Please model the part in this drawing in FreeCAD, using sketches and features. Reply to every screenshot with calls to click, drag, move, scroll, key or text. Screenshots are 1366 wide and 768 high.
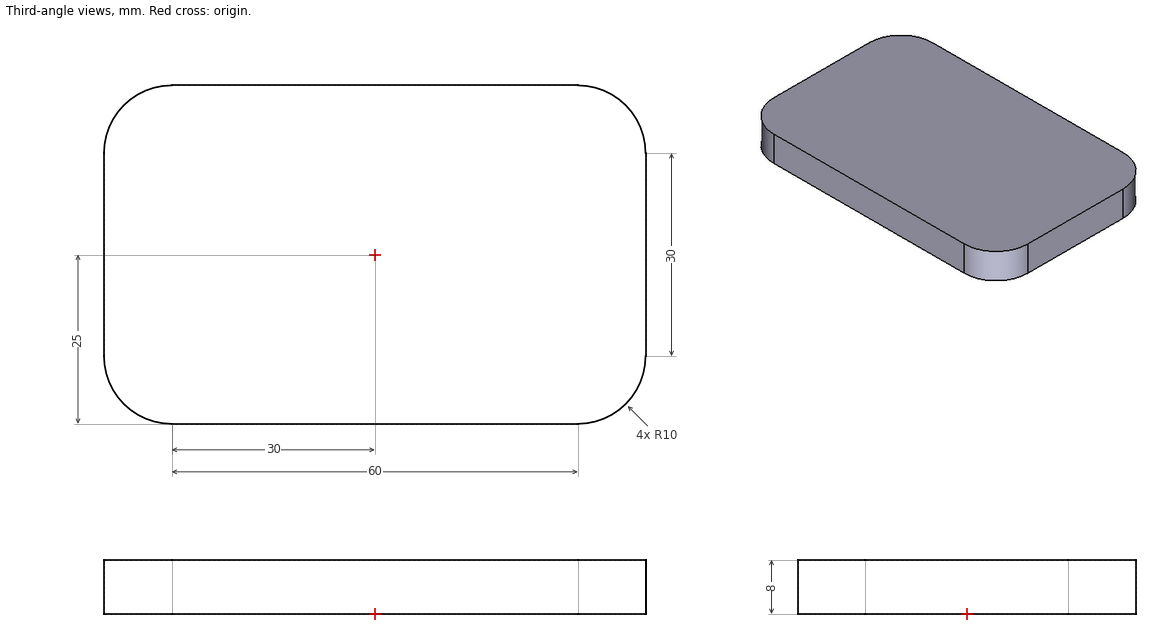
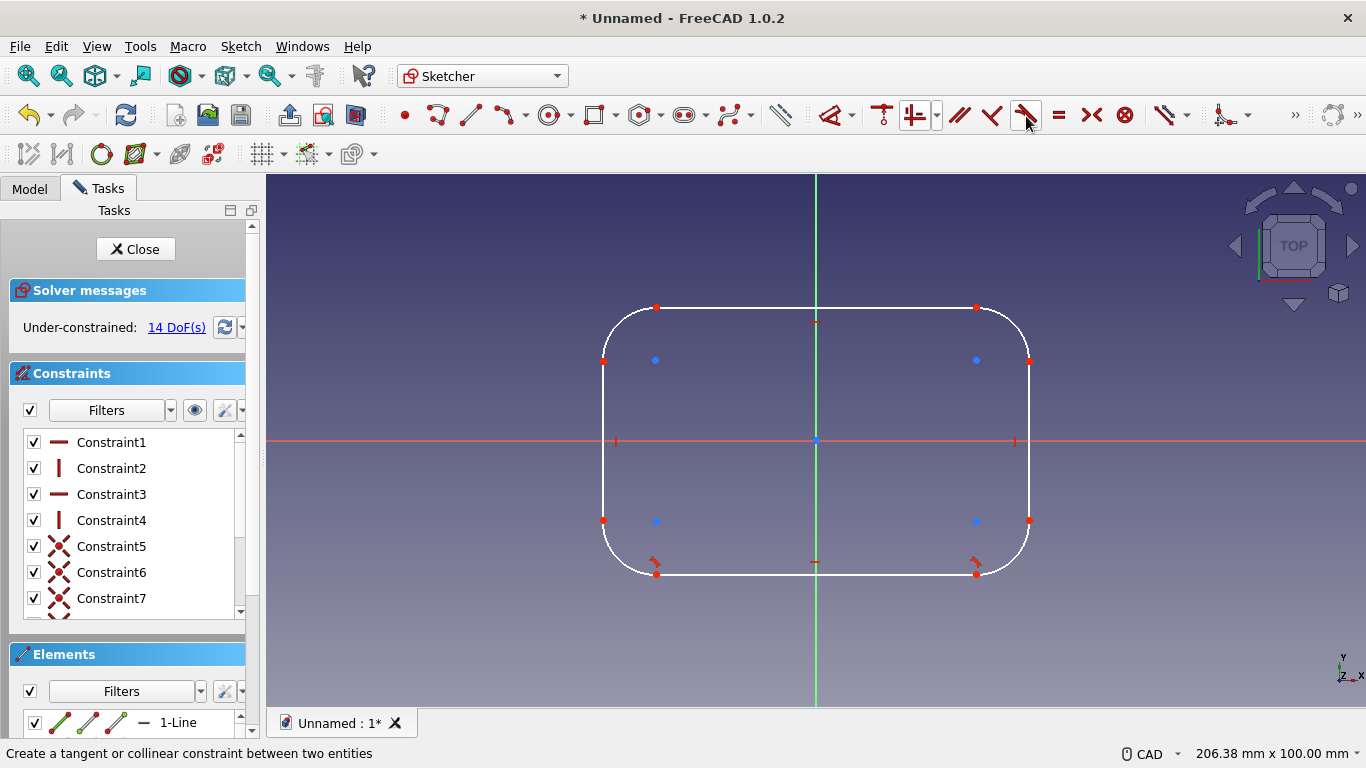
click(1029, 473)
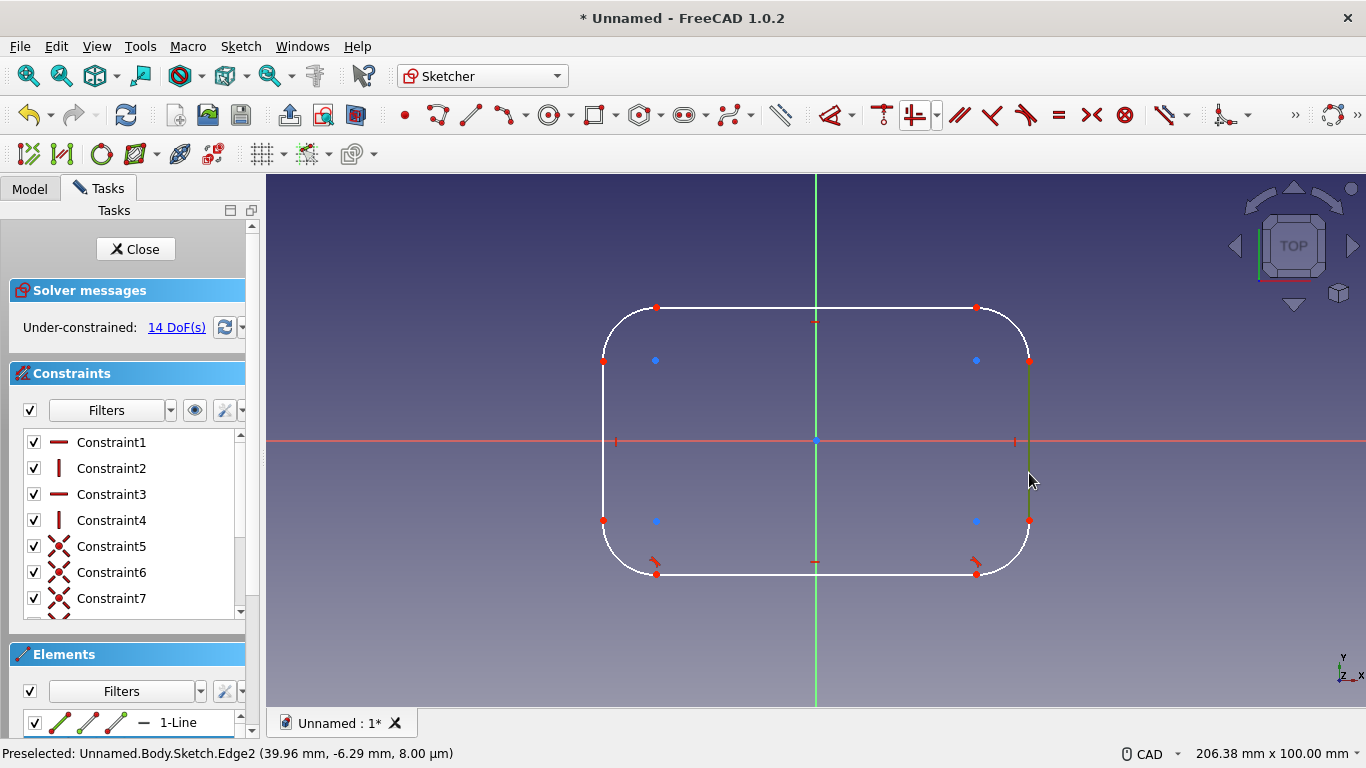
click(1000, 569)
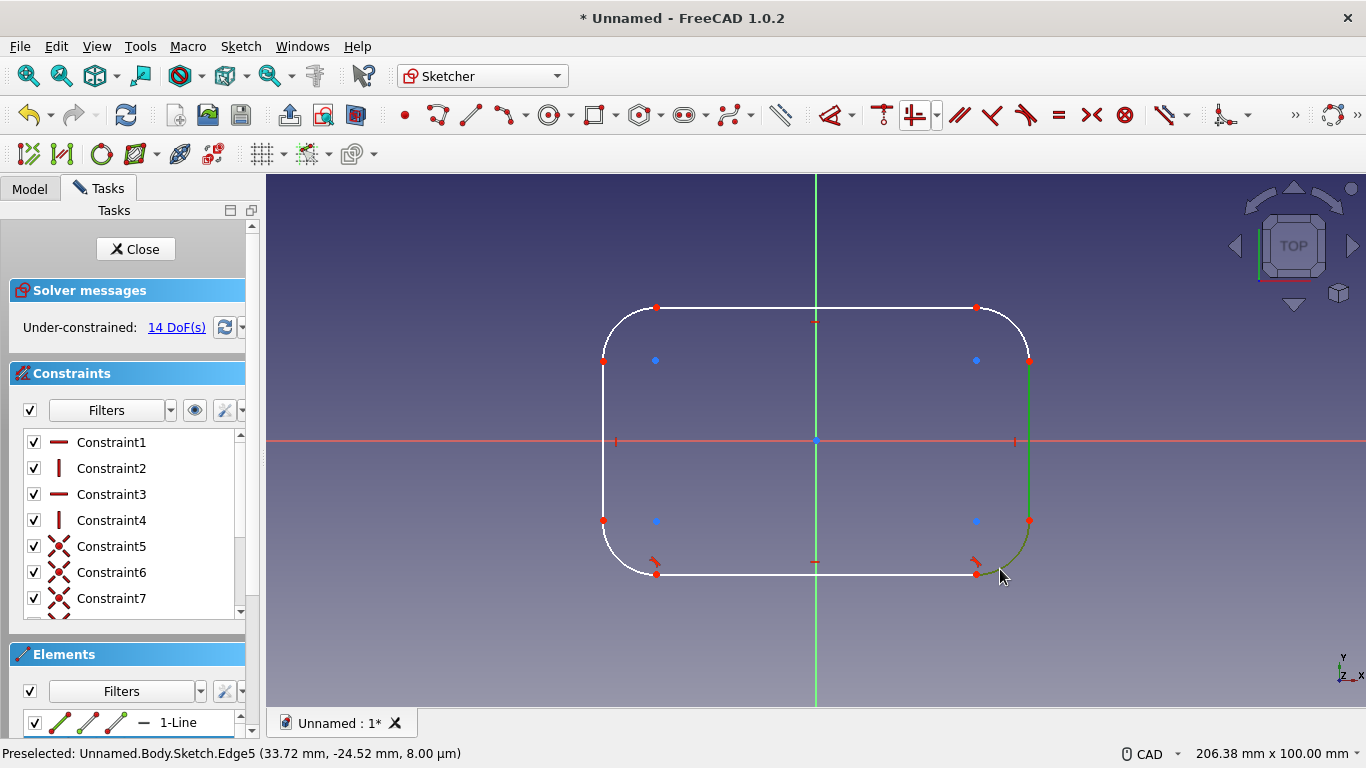
click(1026, 116)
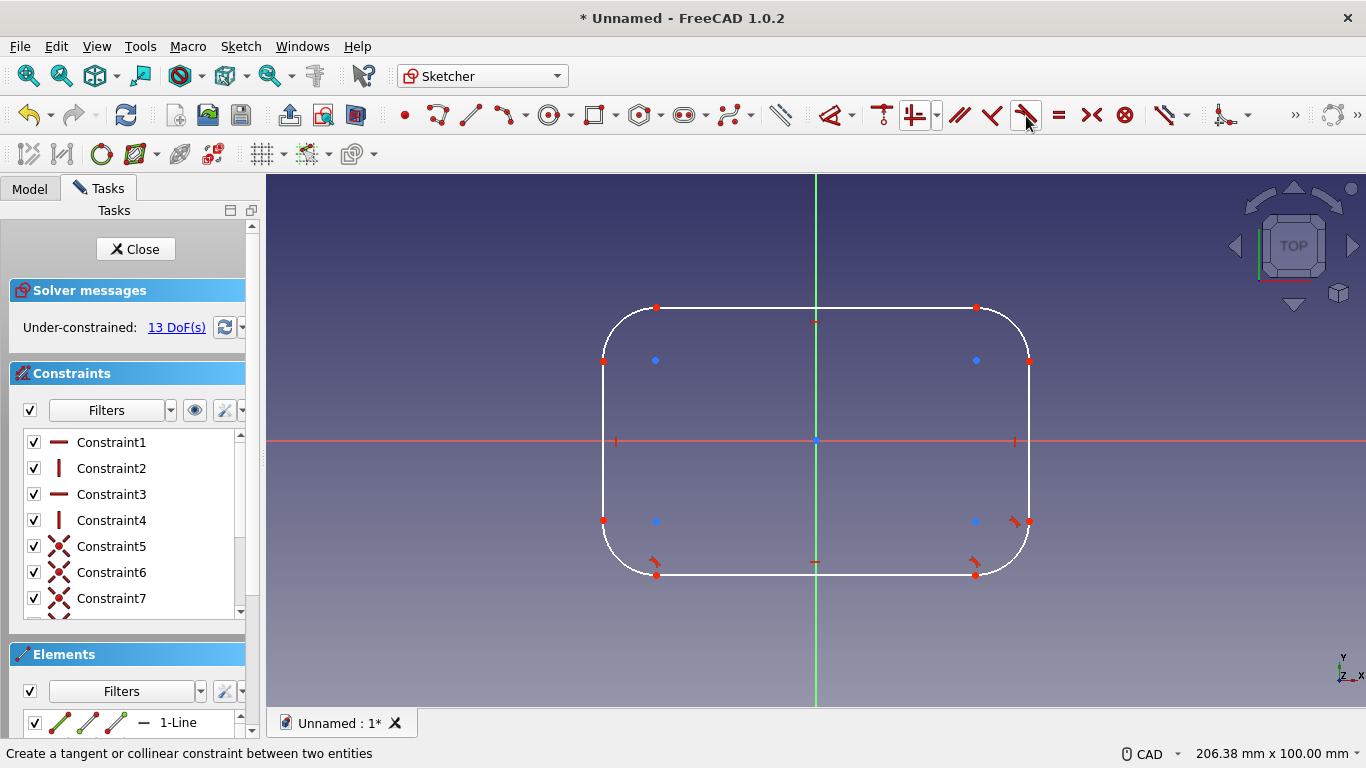
click(1029, 473)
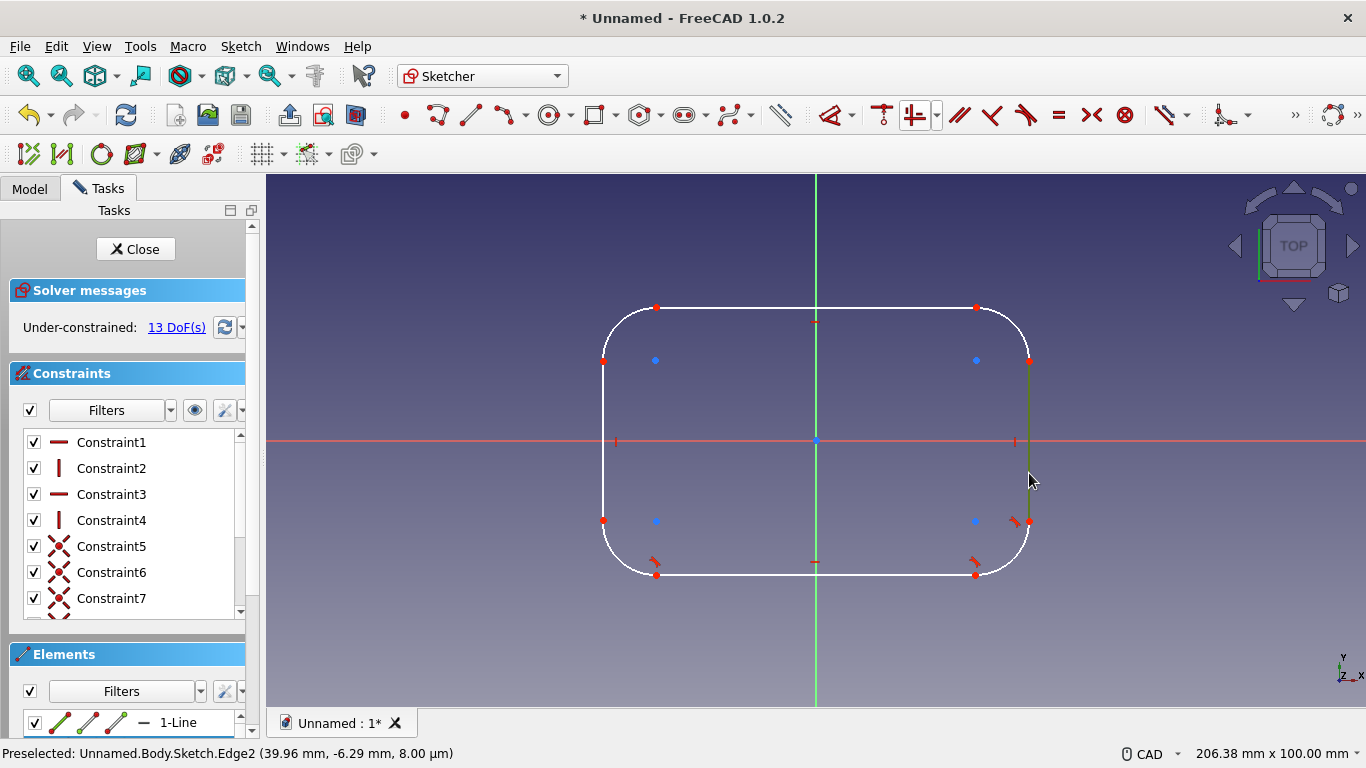
click(1024, 338)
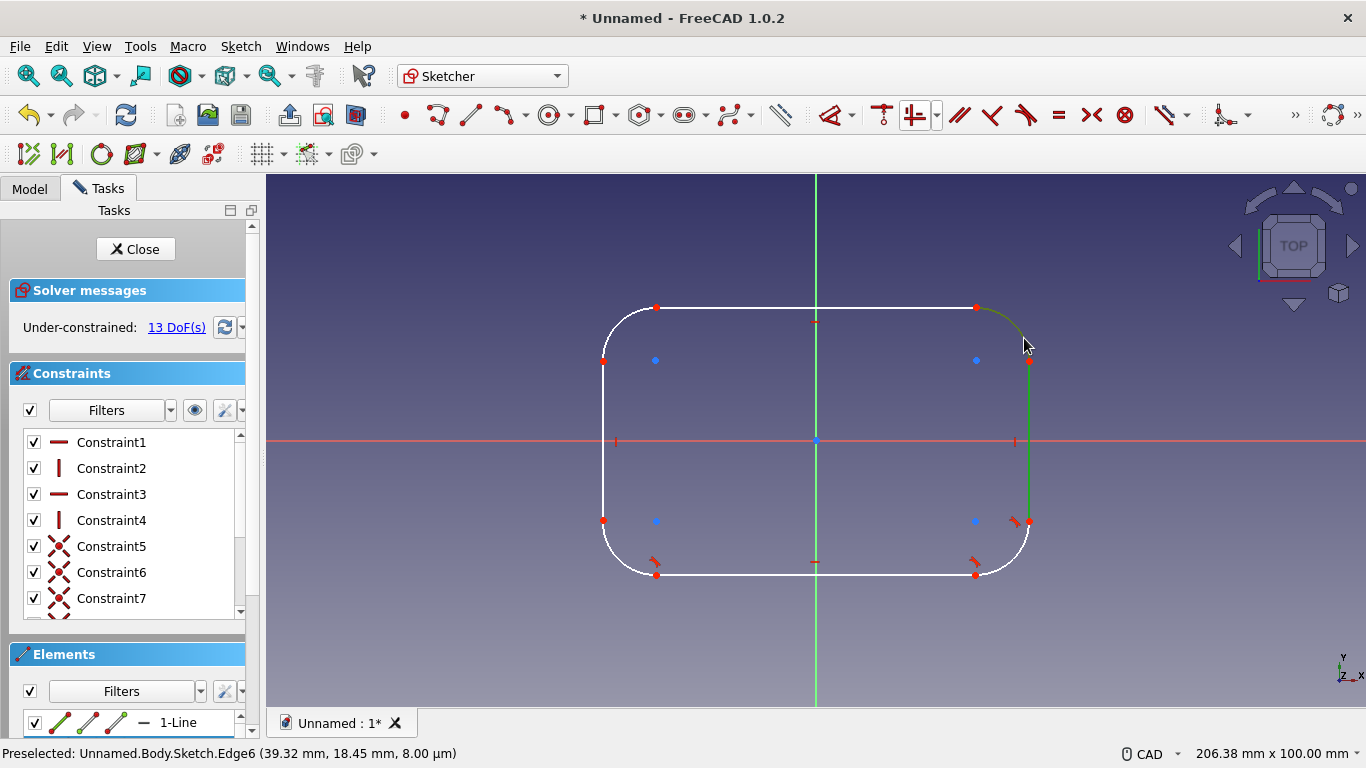
key(t)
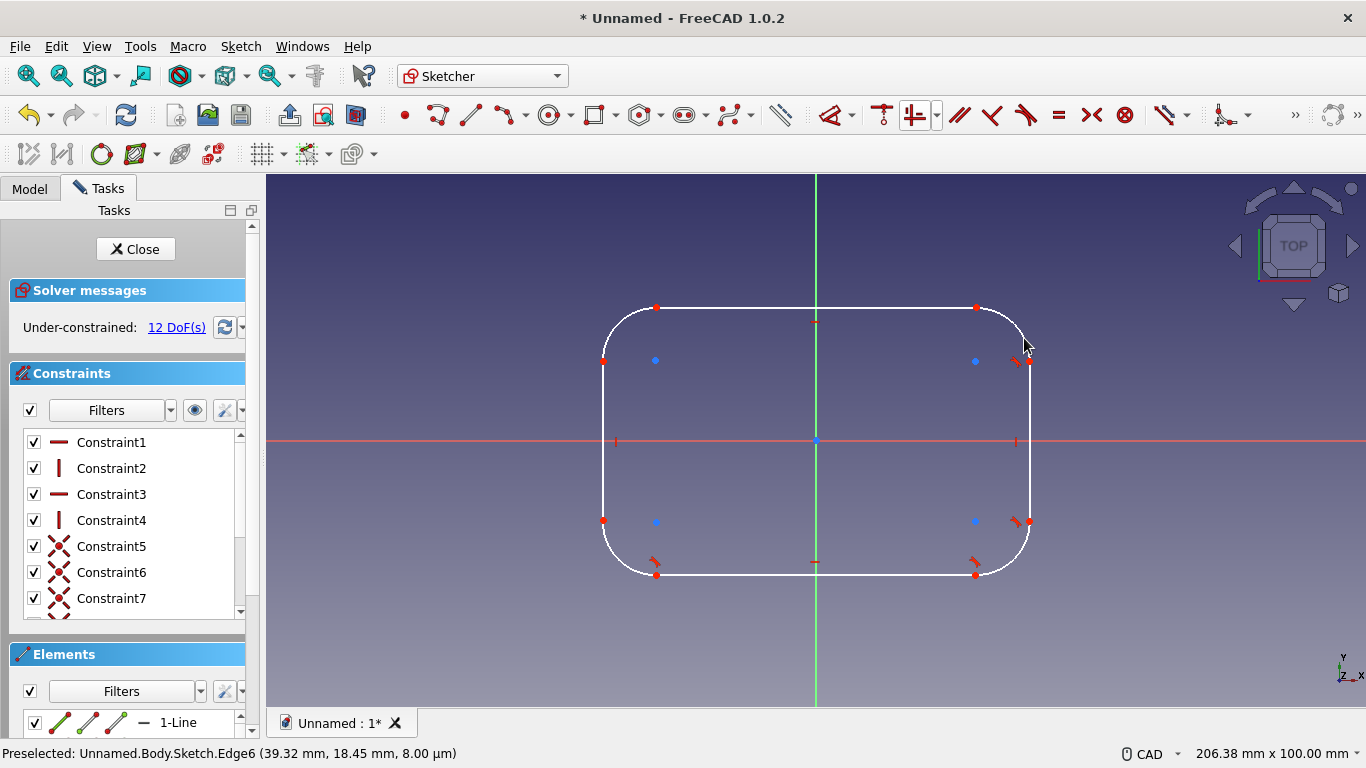
click(880, 308)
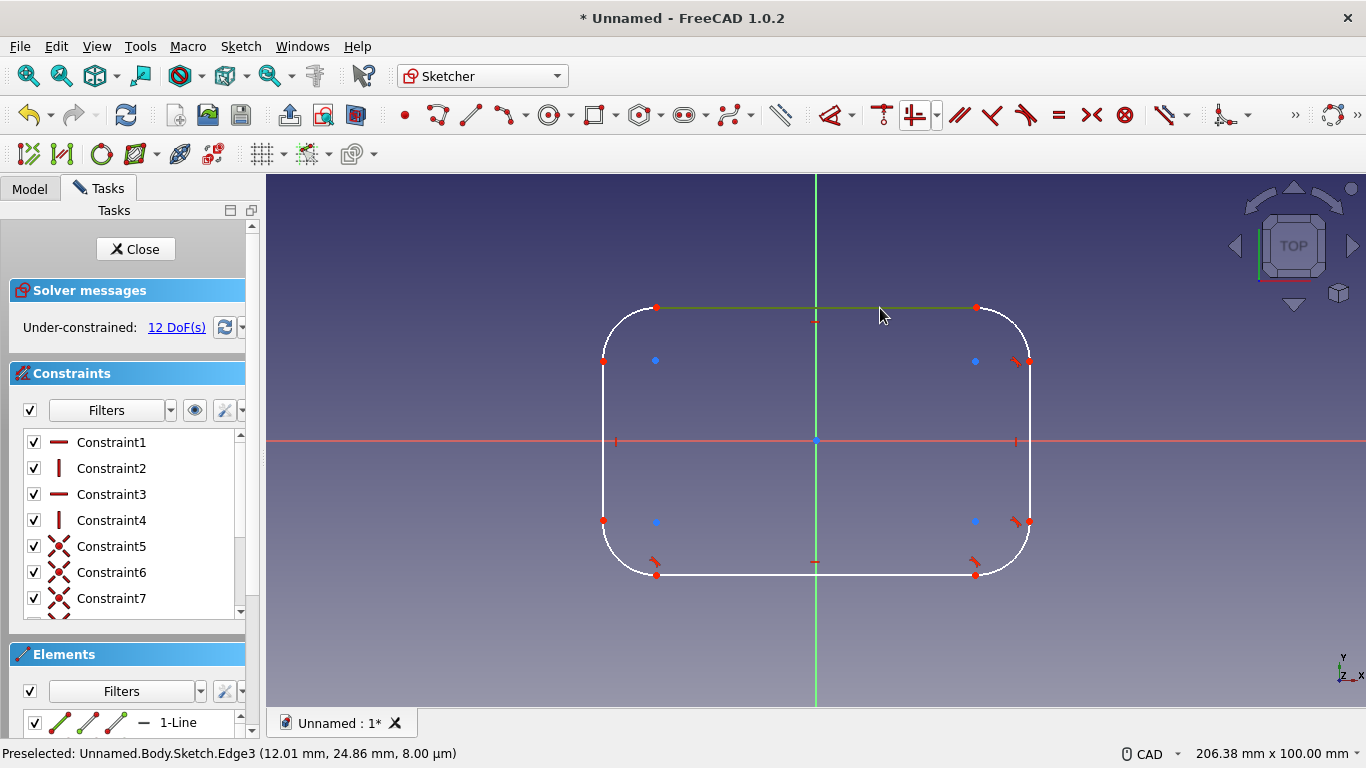
click(1024, 338)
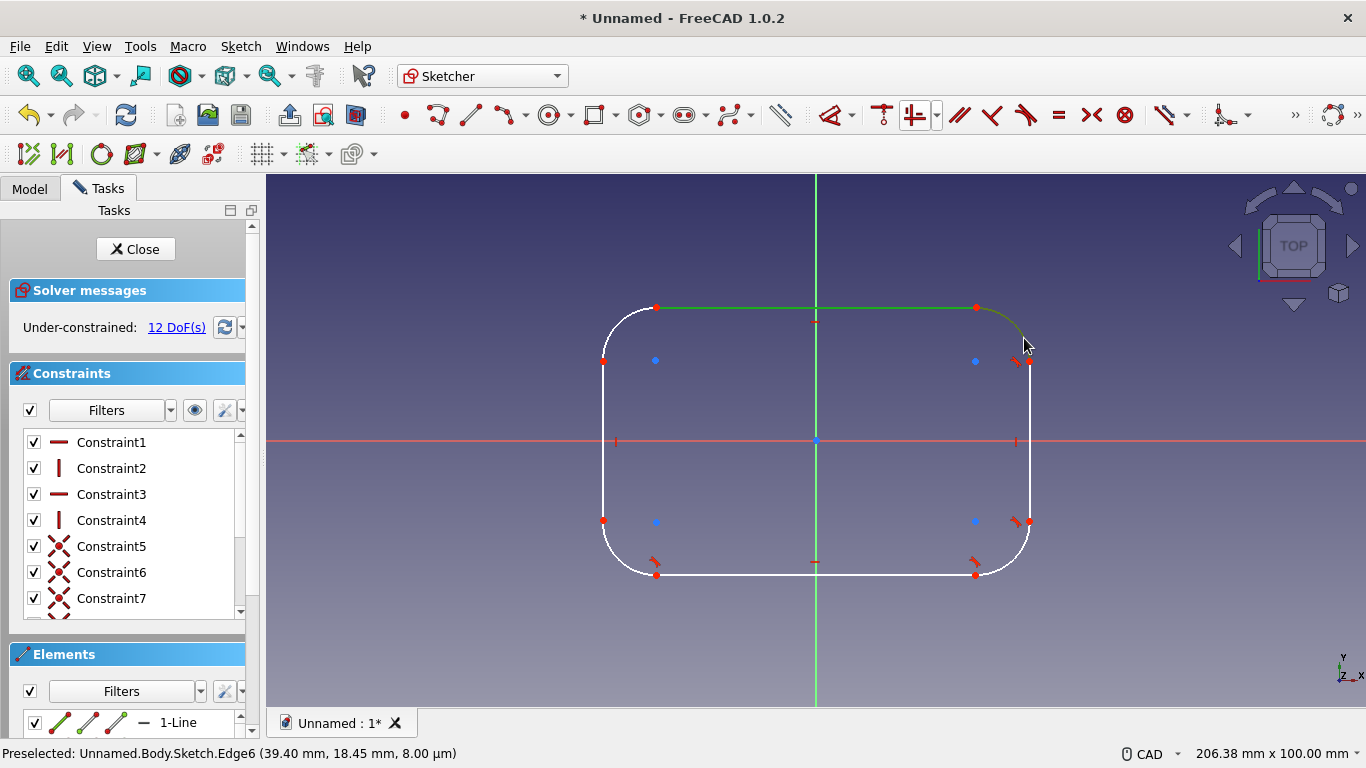
click(1026, 116)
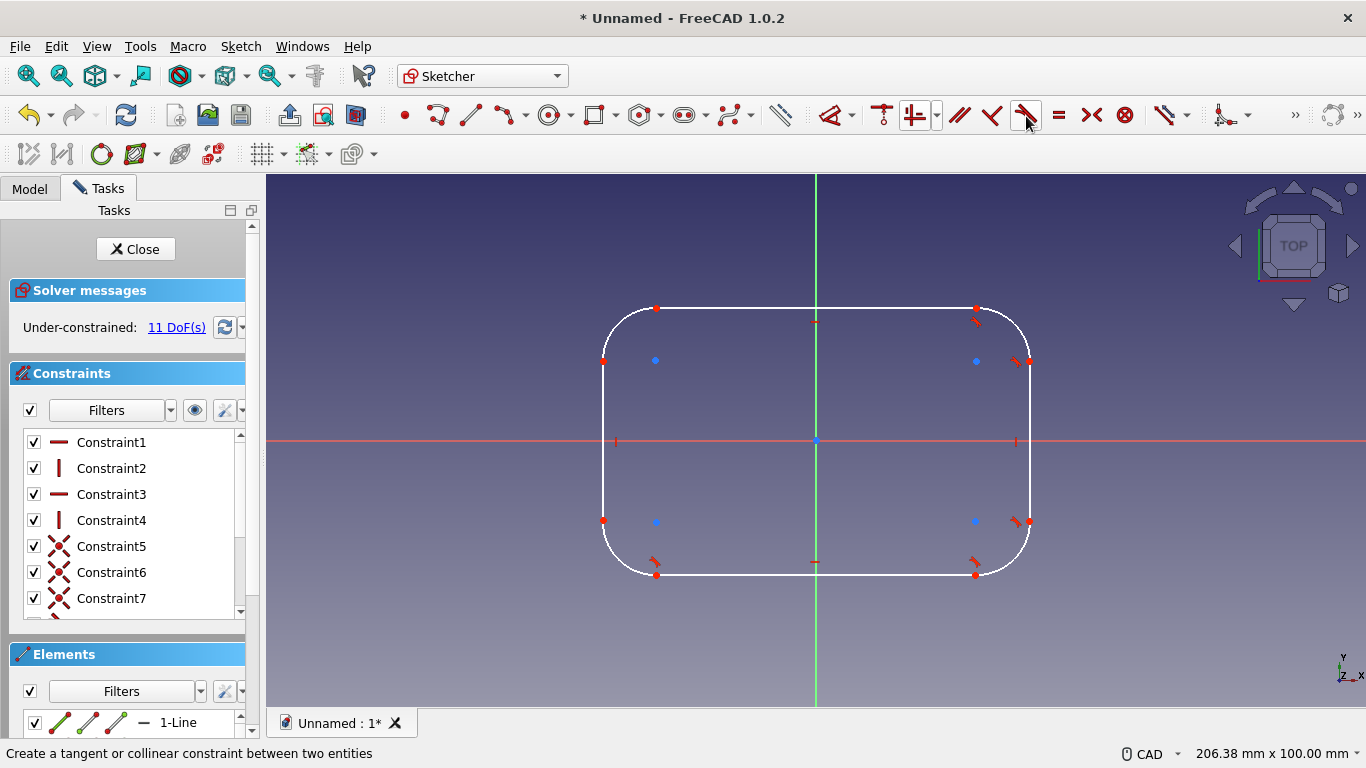
click(880, 308)